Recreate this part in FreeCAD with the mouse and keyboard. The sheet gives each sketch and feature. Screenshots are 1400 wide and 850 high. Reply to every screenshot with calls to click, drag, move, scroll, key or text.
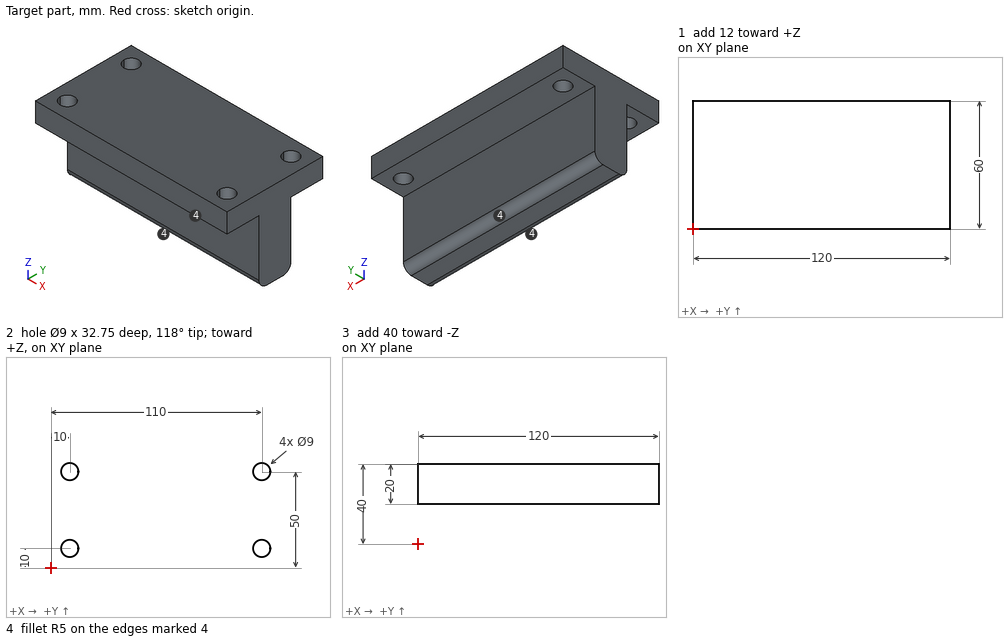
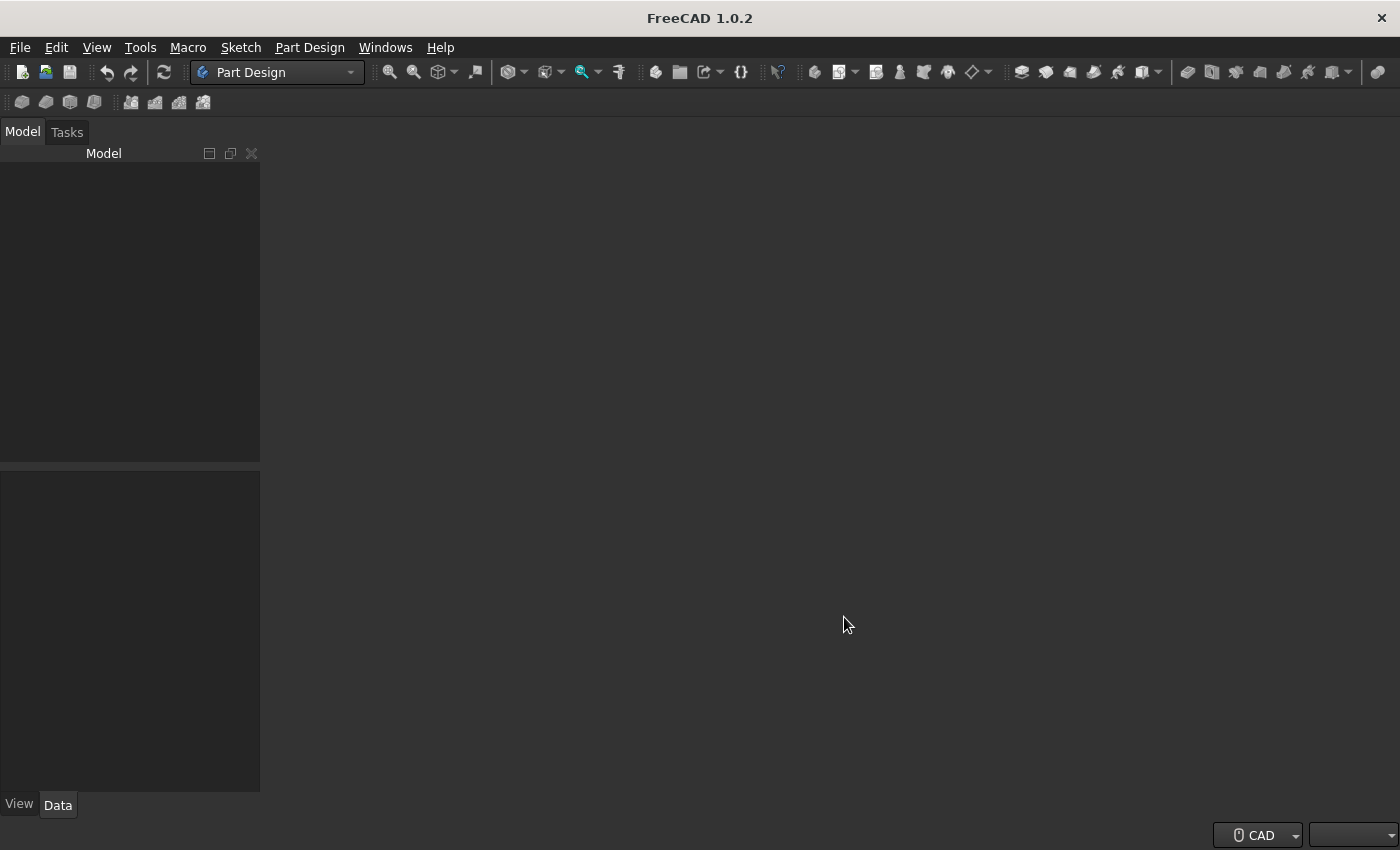
click(22, 72)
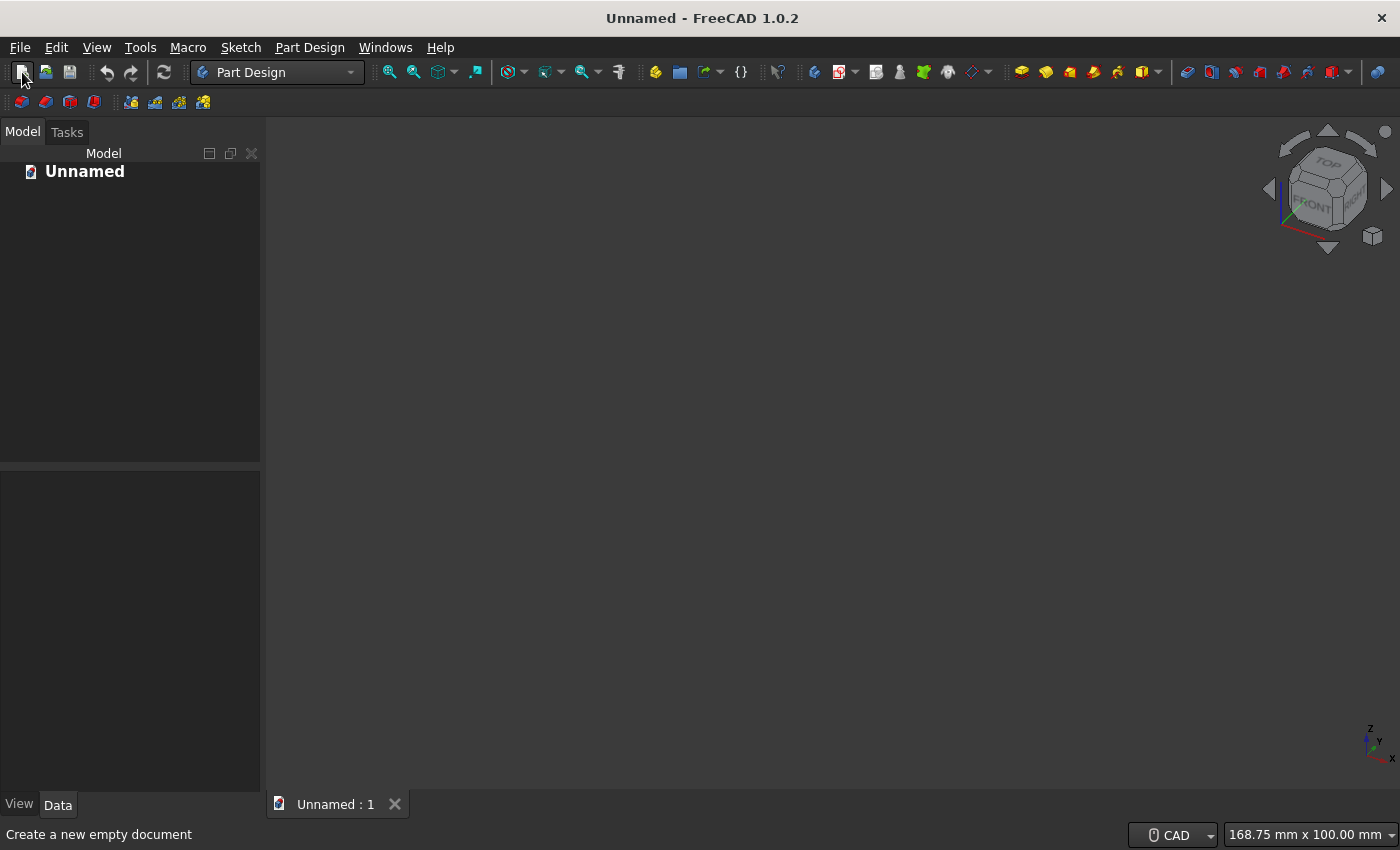
click(840, 72)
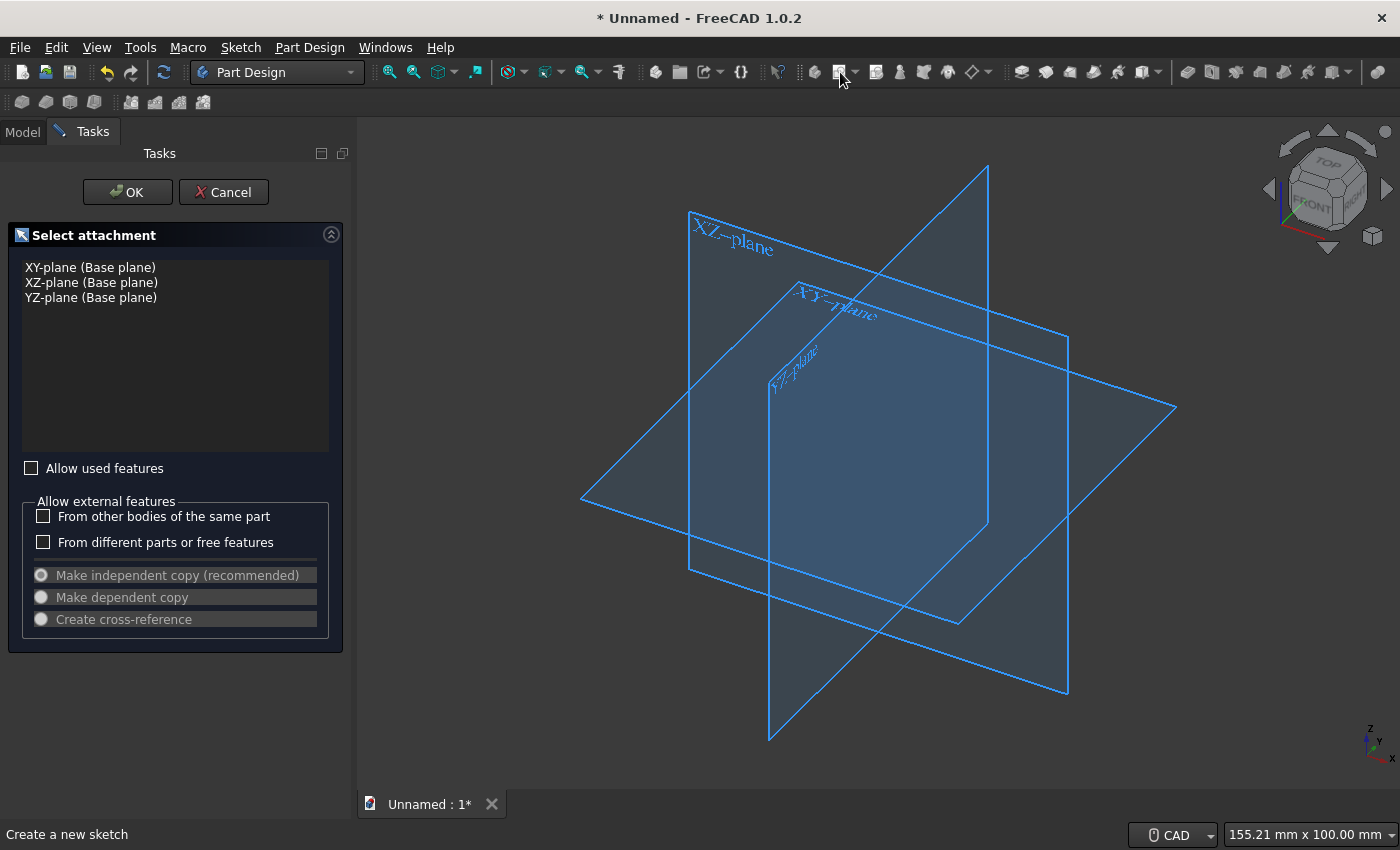
click(82, 268)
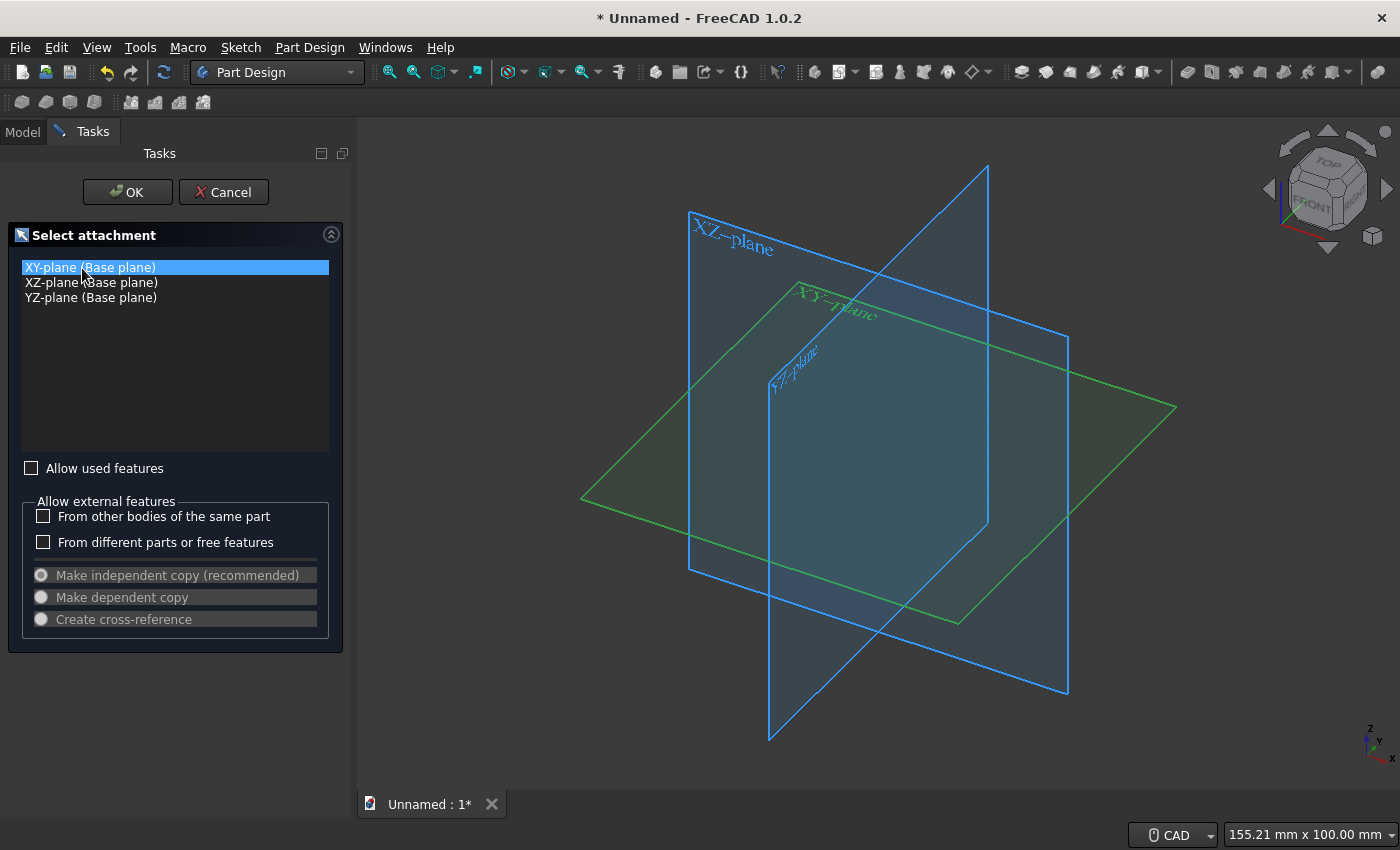
click(128, 192)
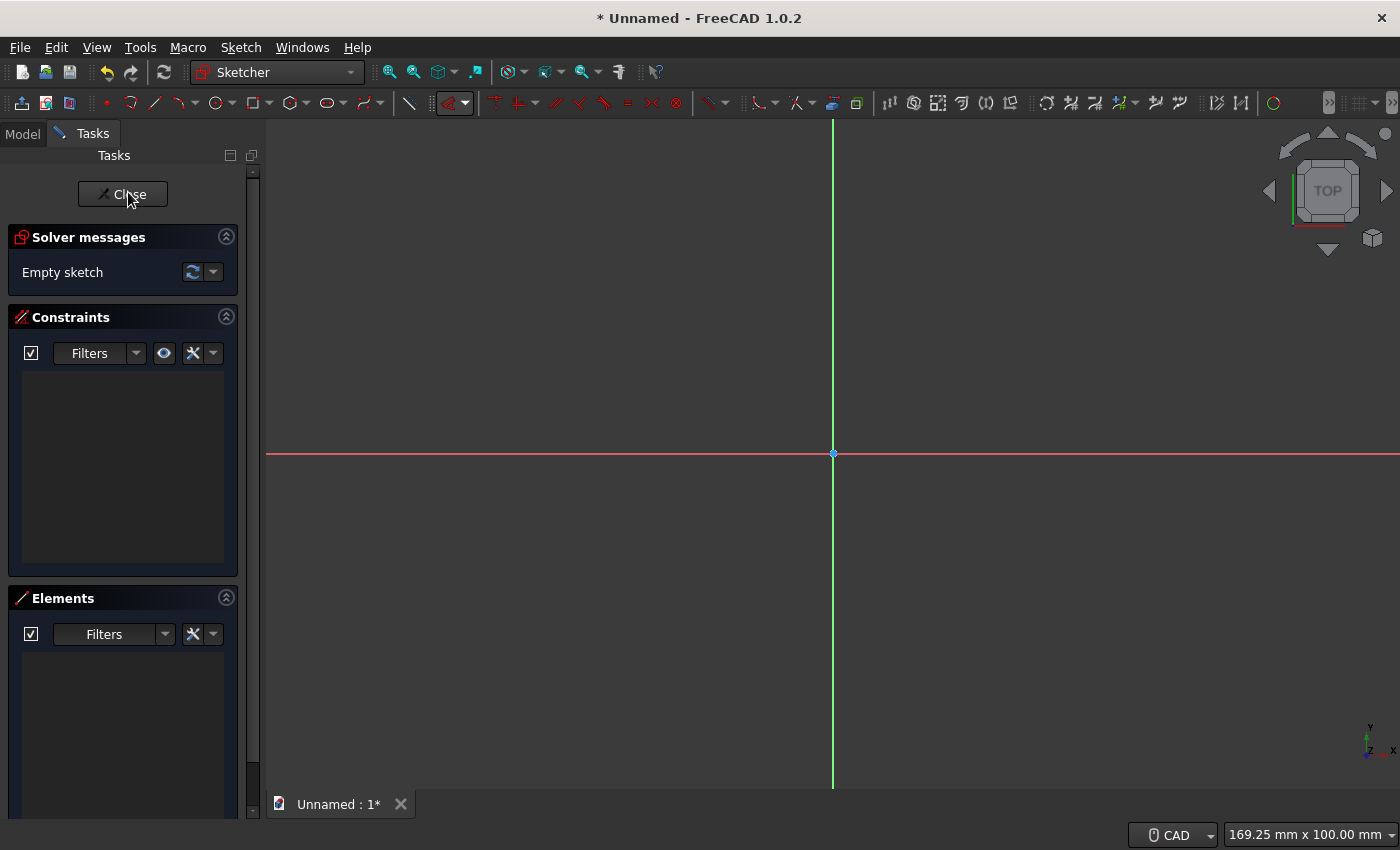
scroll(294, 761, down, 2)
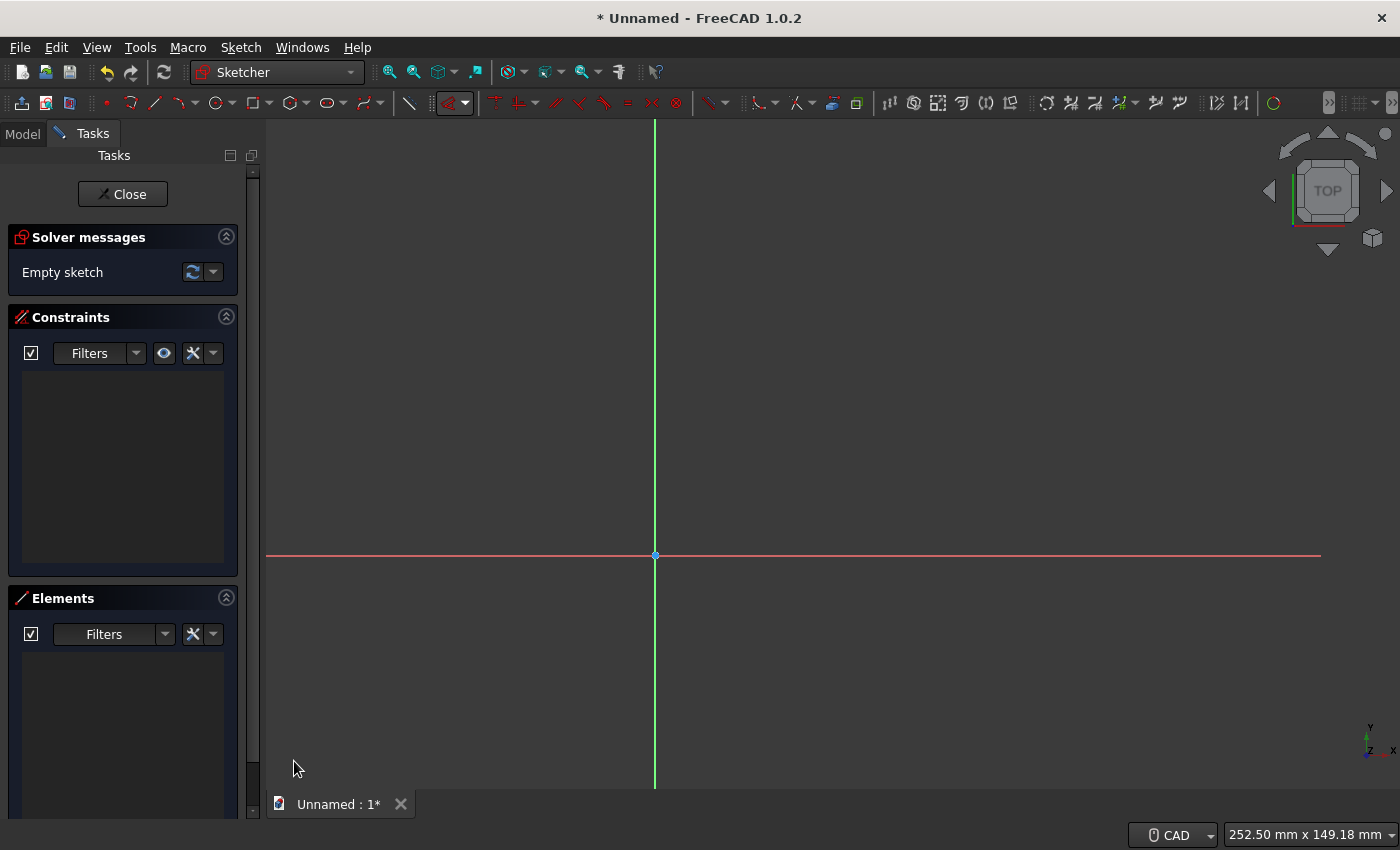
click(254, 104)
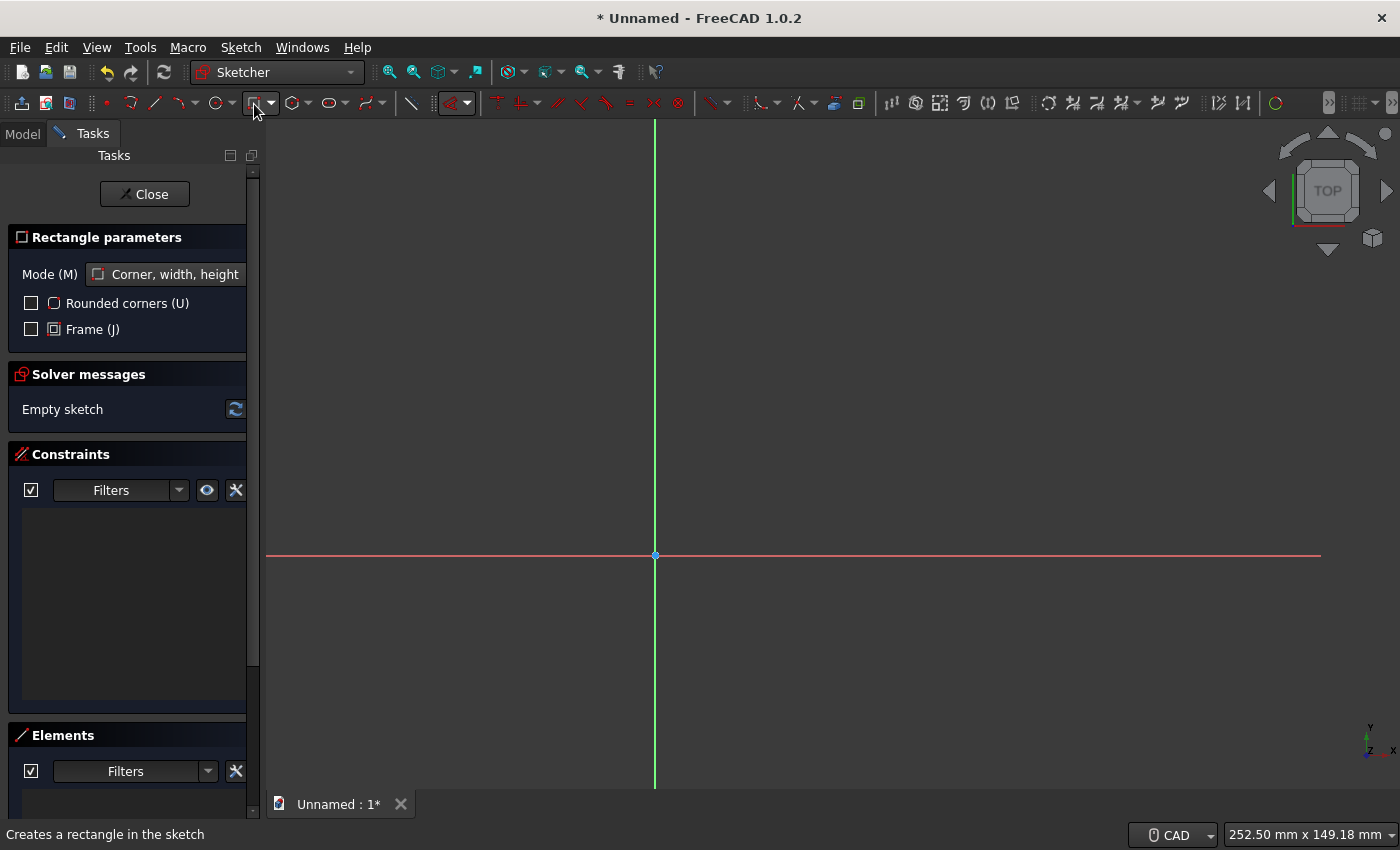
click(655, 556)
click(1194, 286)
key(Escape)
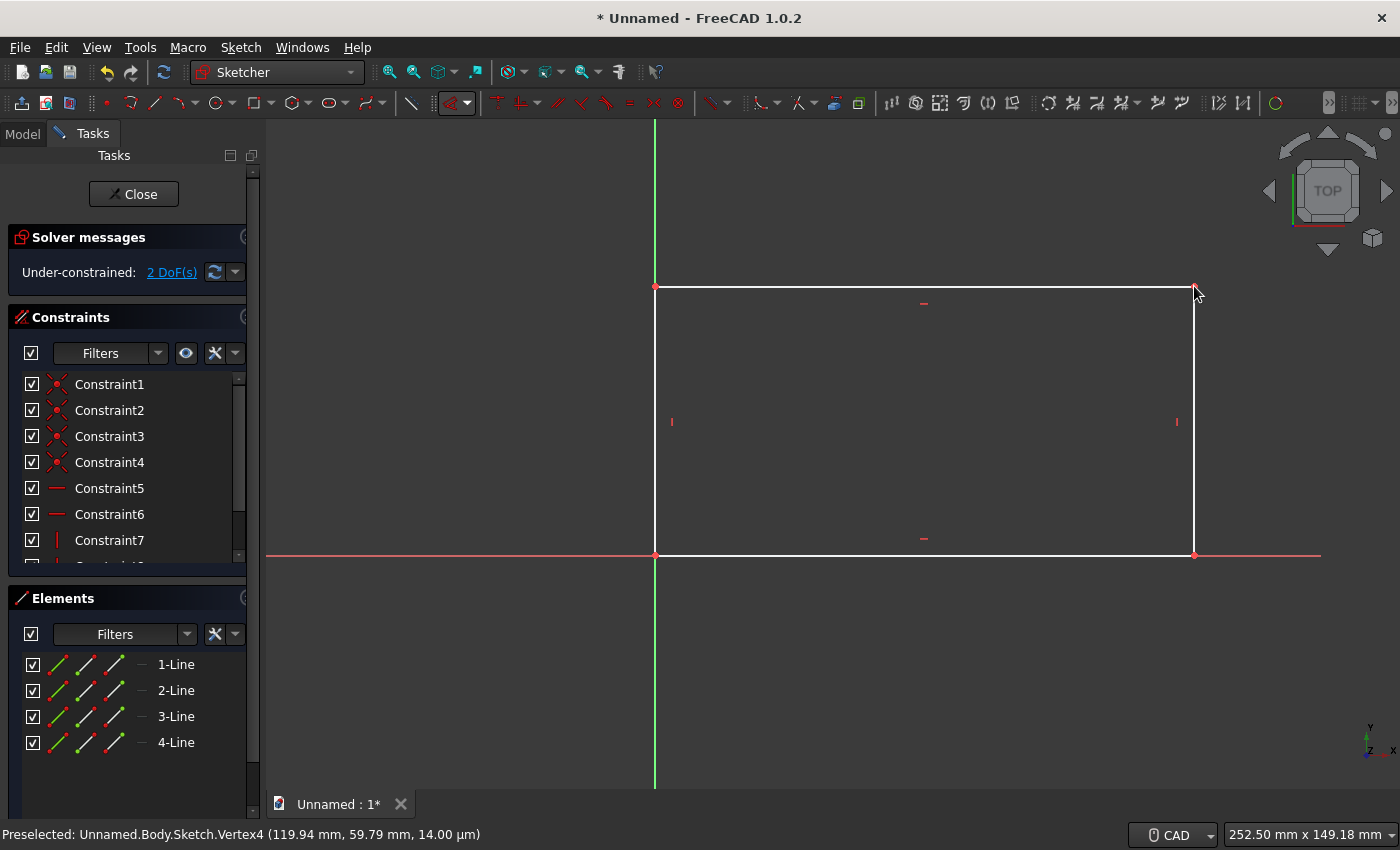
click(1194, 475)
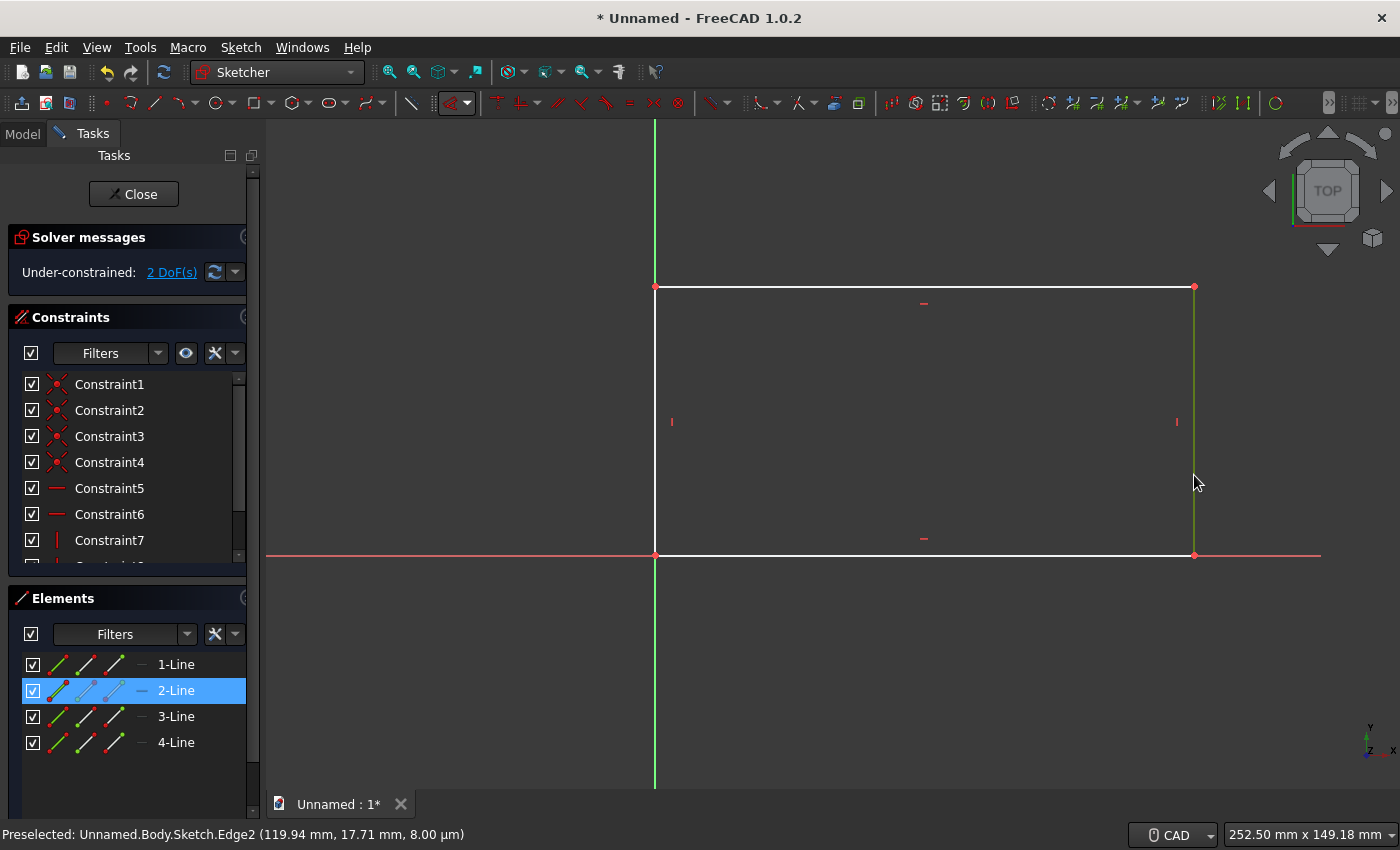
key(i)